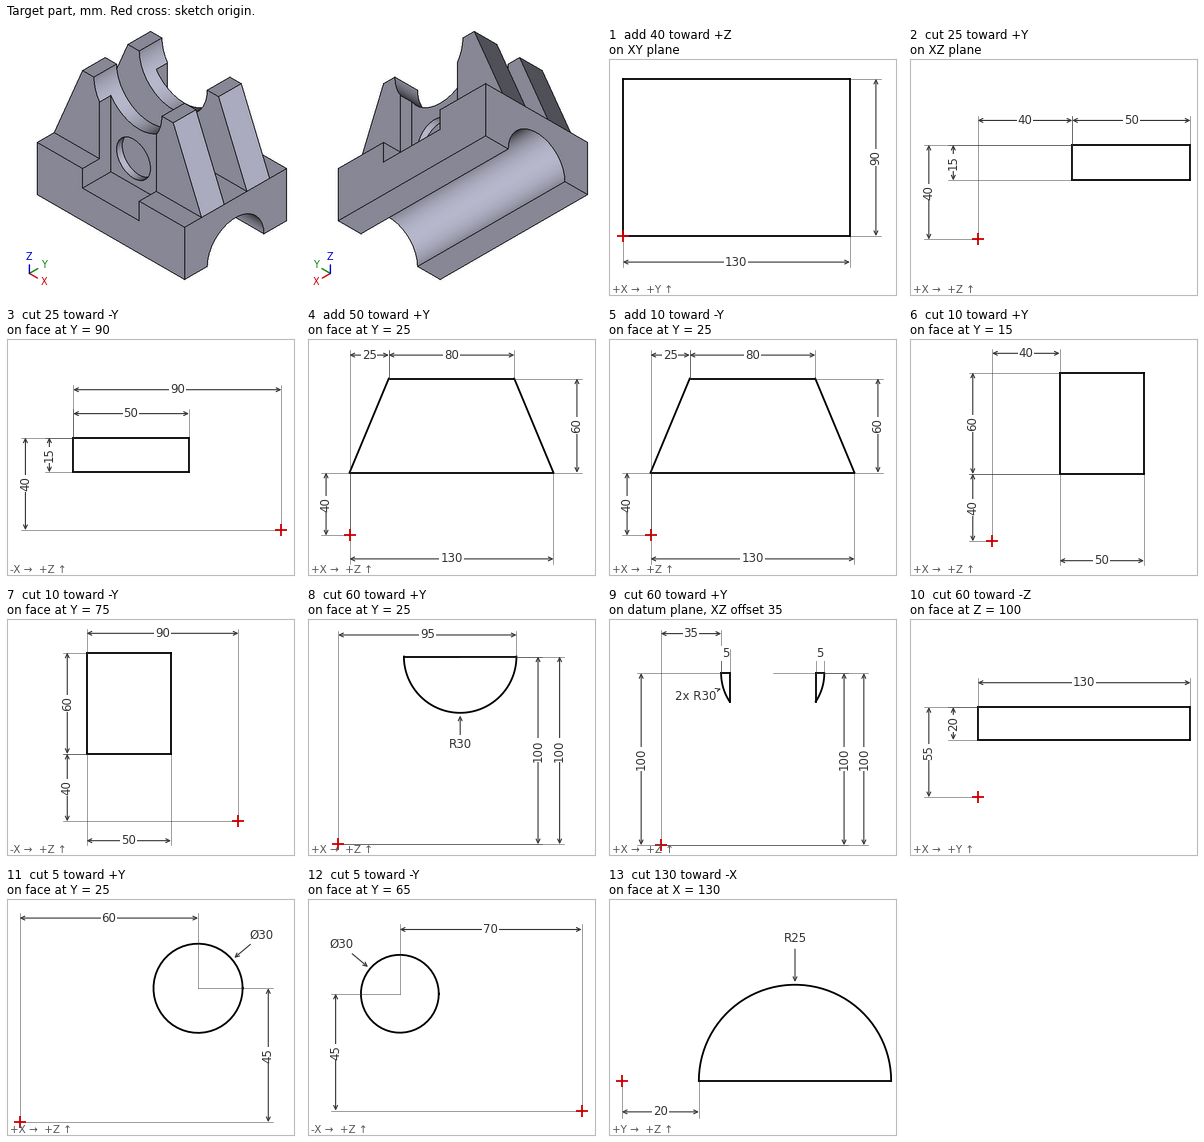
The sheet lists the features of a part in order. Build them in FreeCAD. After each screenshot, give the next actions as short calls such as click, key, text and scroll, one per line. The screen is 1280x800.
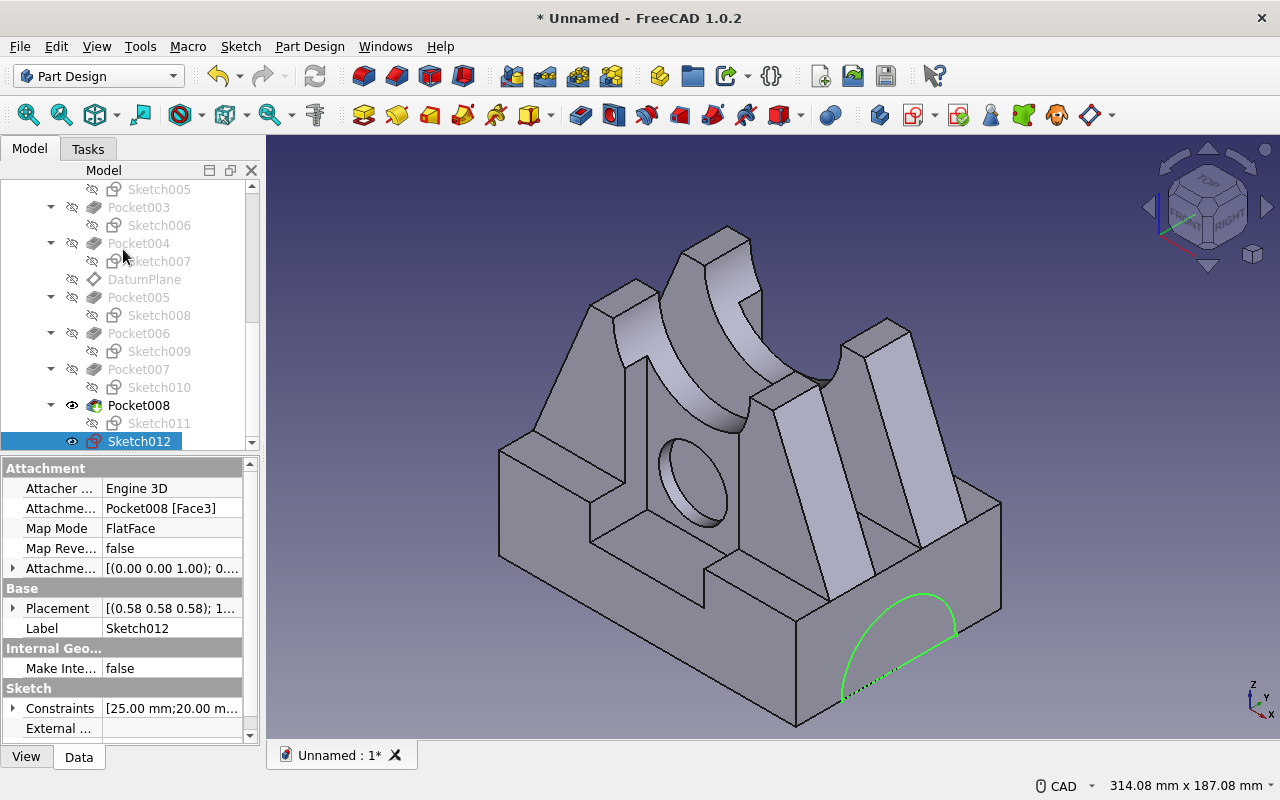
click(581, 116)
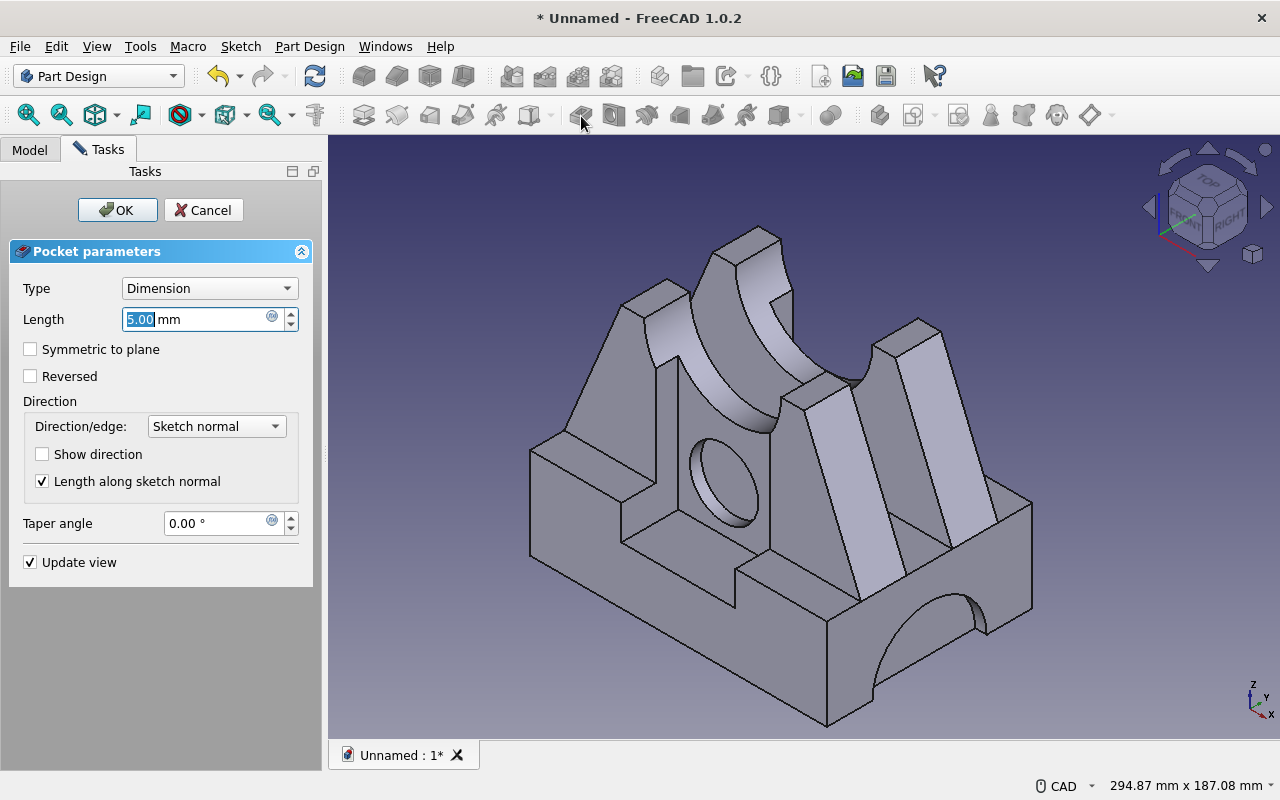
text(130)
key(Tab)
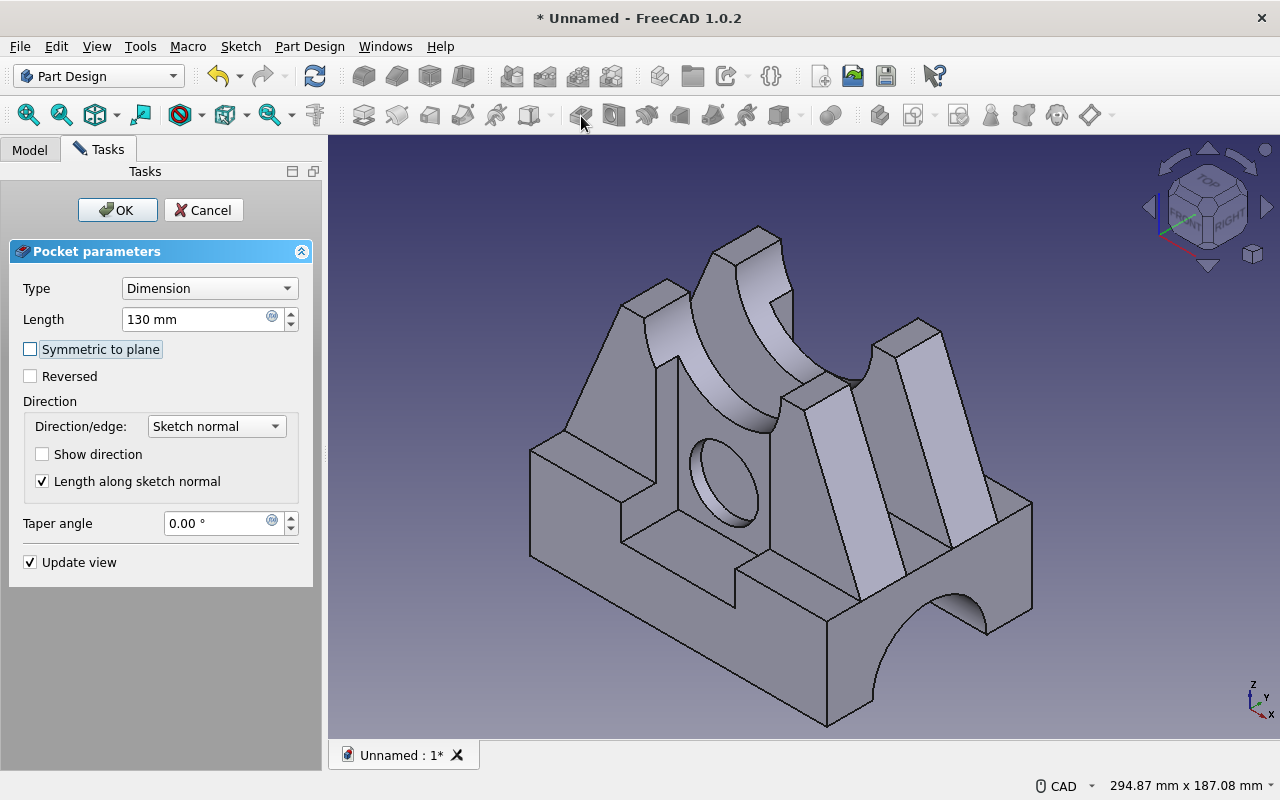
click(118, 210)